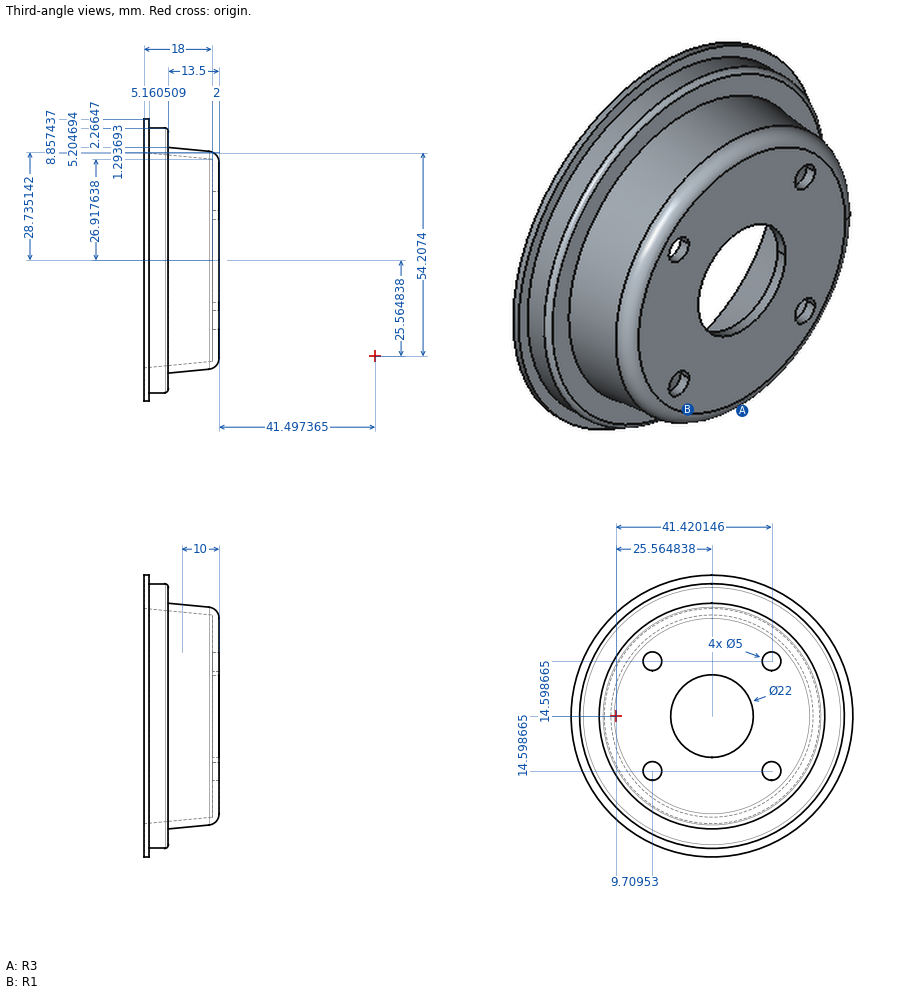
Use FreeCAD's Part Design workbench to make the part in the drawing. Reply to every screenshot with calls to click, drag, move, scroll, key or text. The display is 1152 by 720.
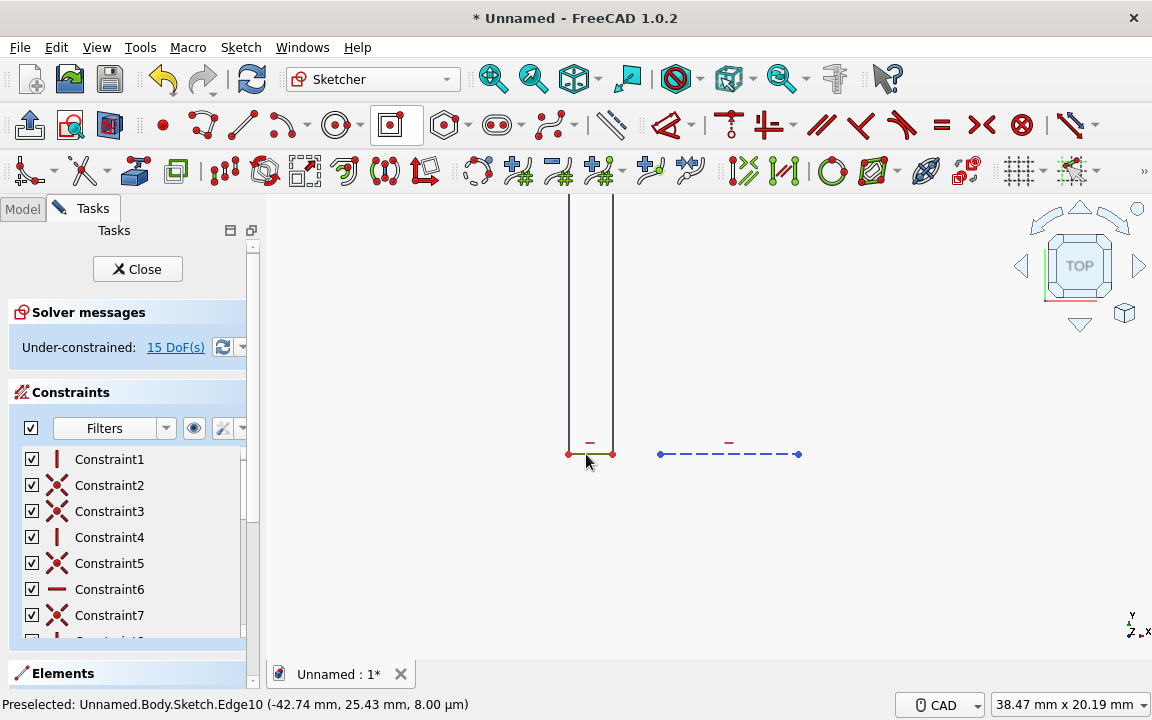
click(694, 126)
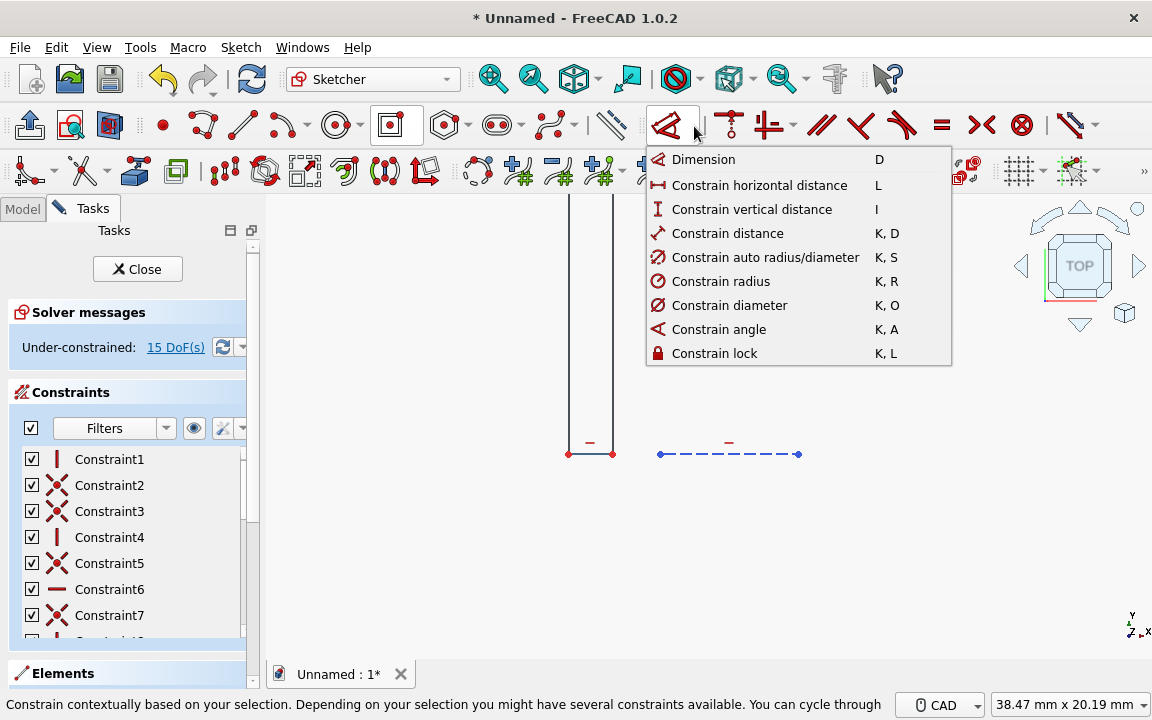
click(799, 185)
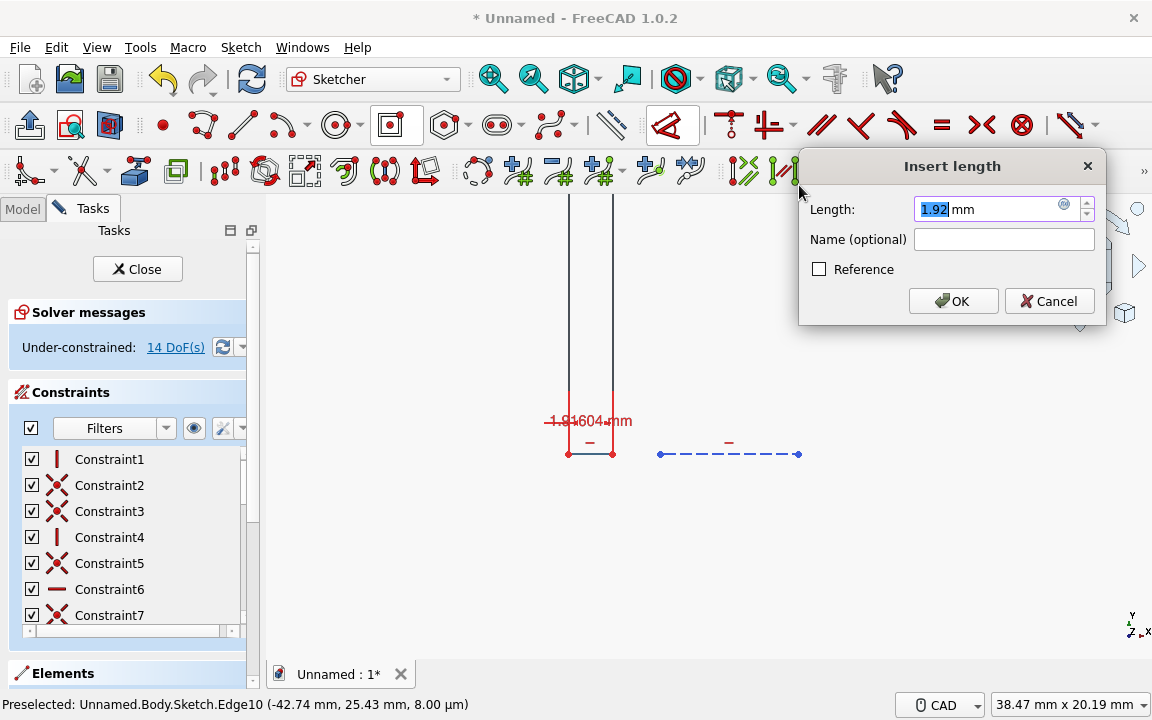
text(2)
key(Return)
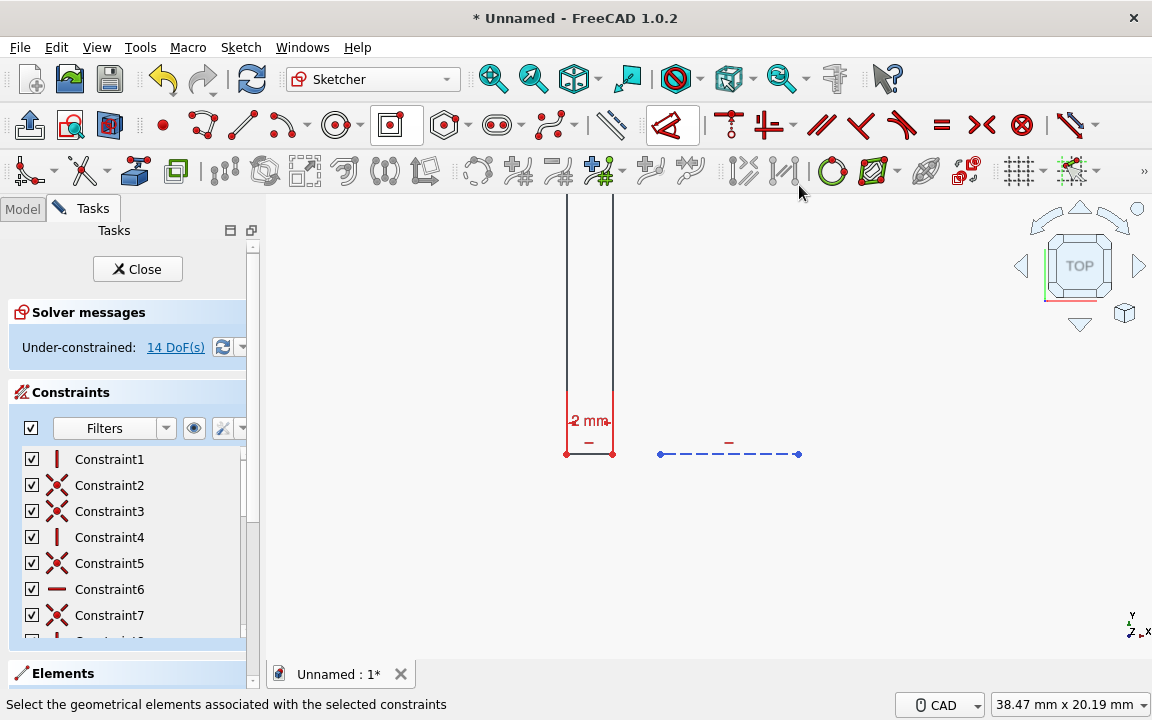
scroll(584, 455, down, 8)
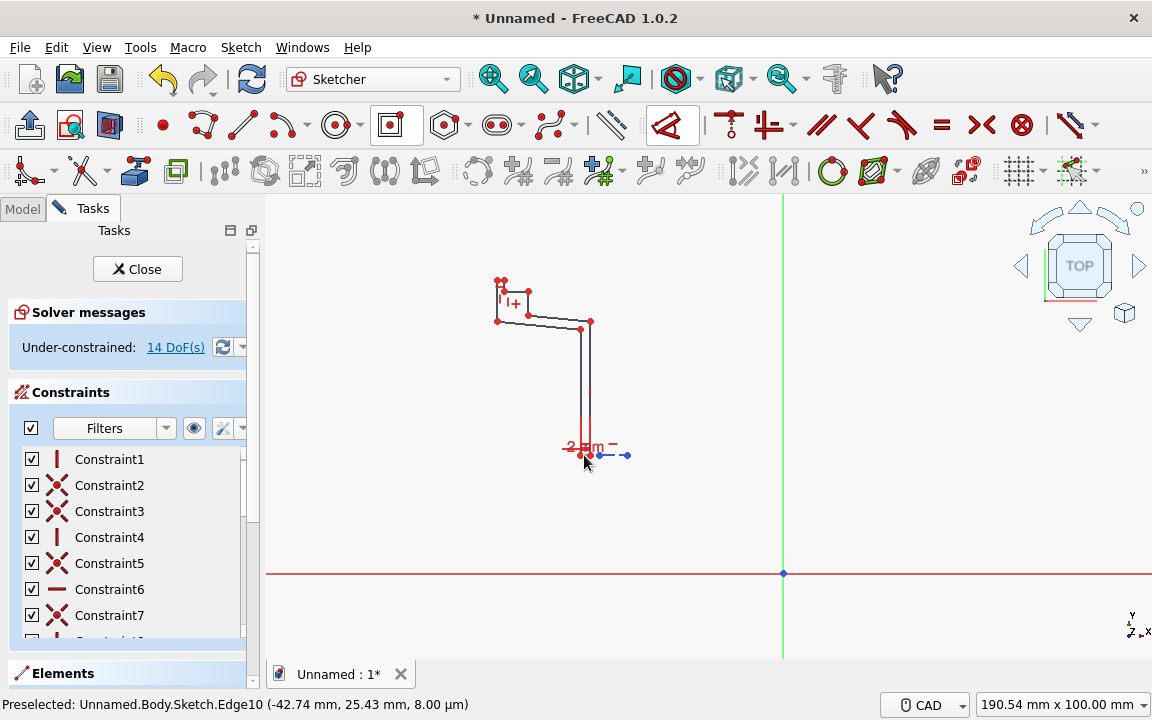
scroll(522, 324, up, 2)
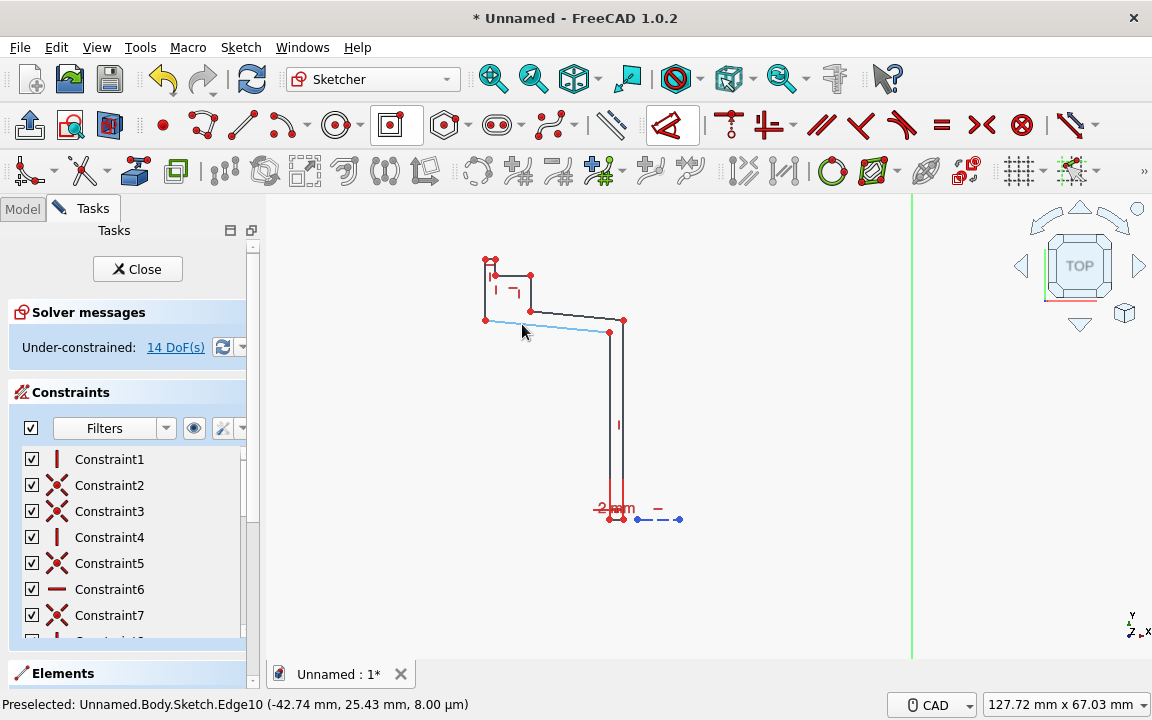
click(522, 324)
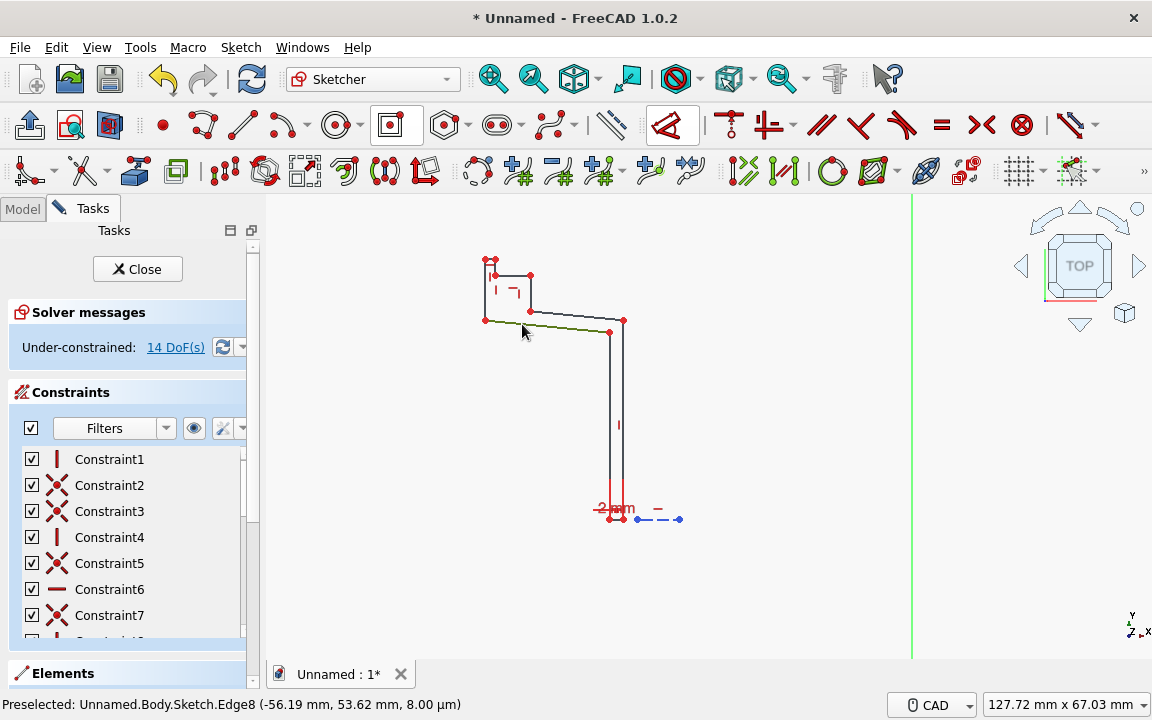
key(l)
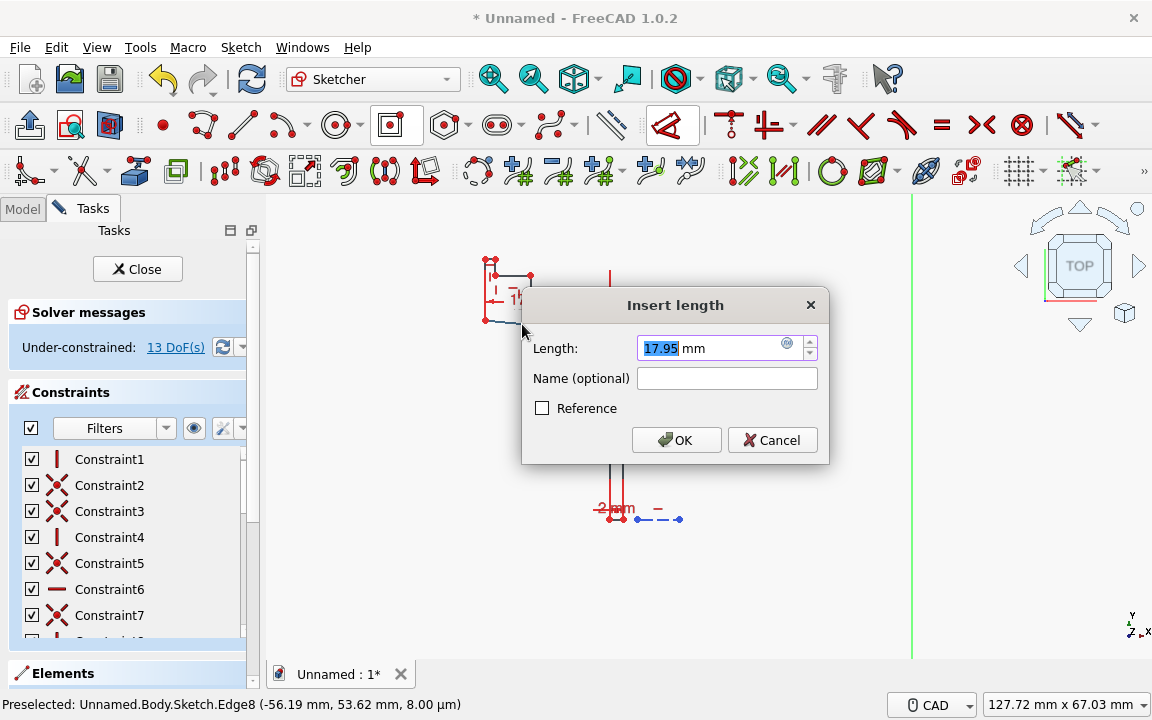
text(18)
key(Return)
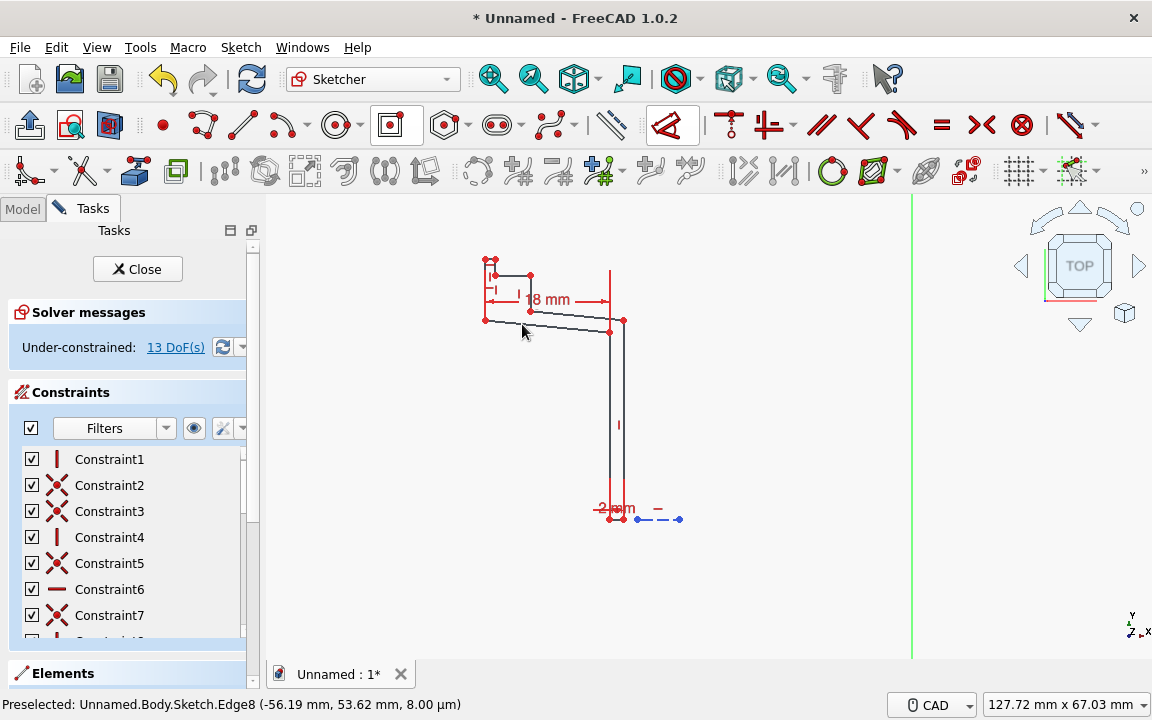
click(596, 318)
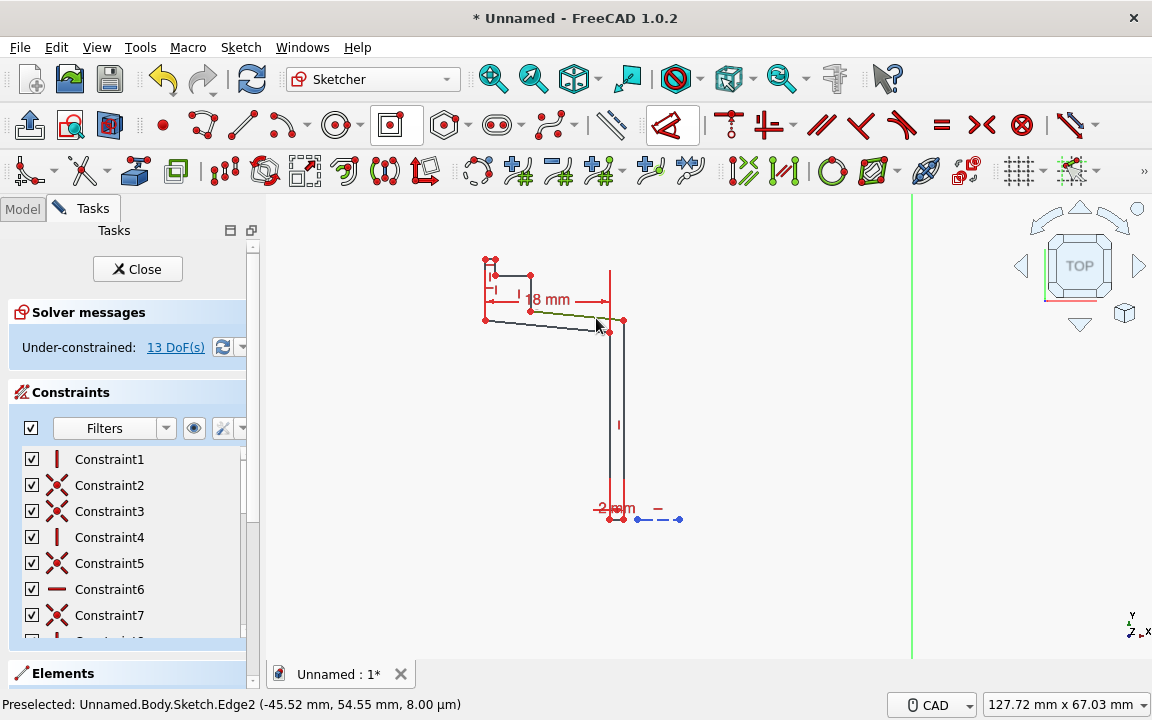
key(l)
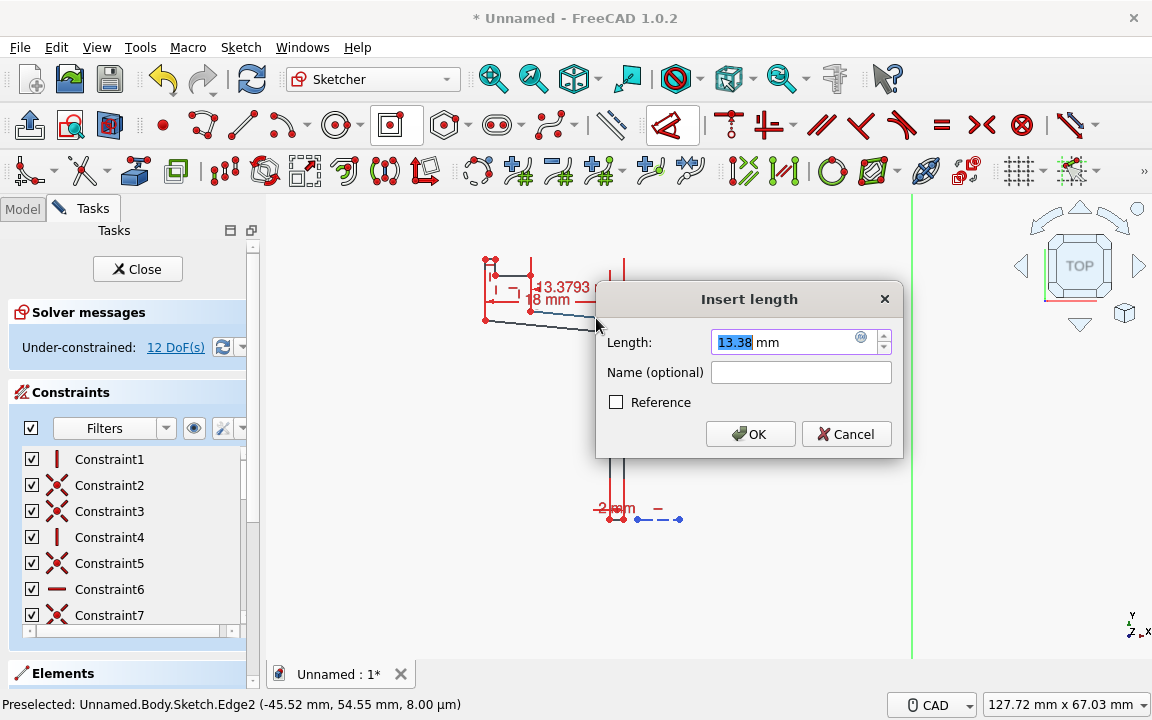
text(13.5)
key(Return)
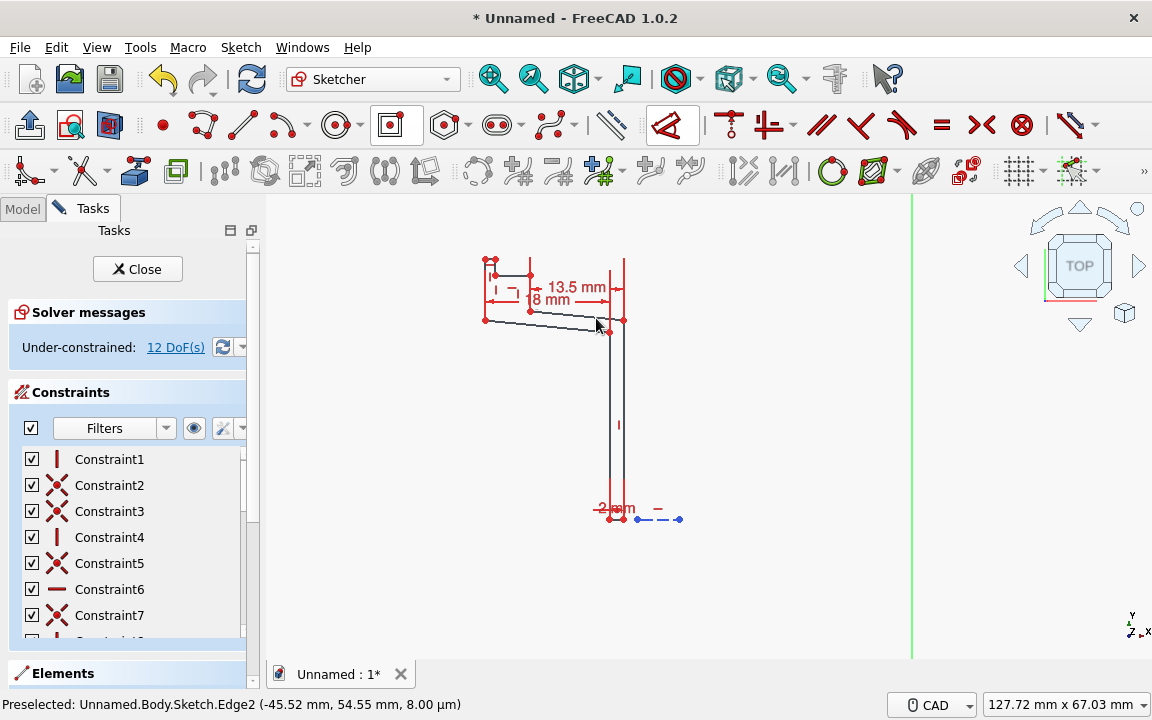
scroll(495, 267, up, 5)